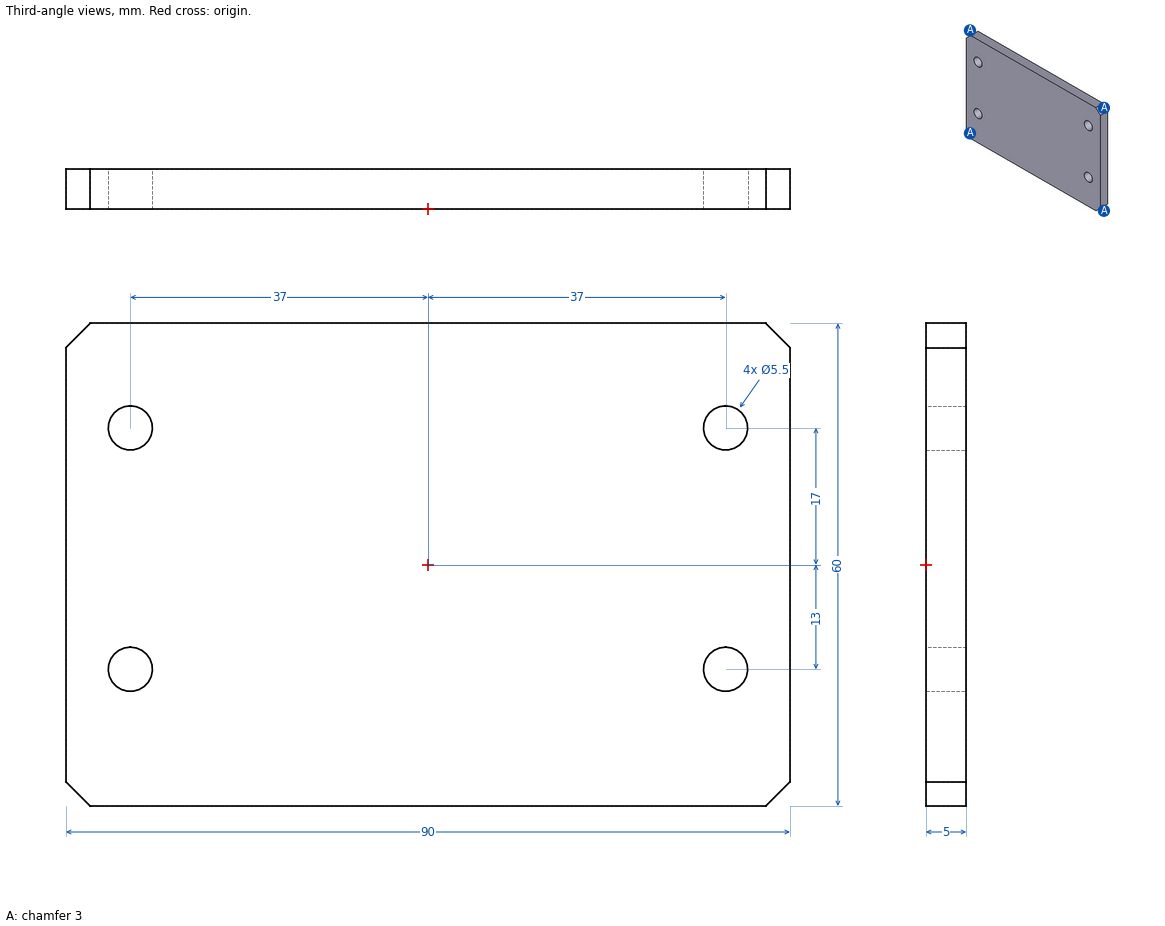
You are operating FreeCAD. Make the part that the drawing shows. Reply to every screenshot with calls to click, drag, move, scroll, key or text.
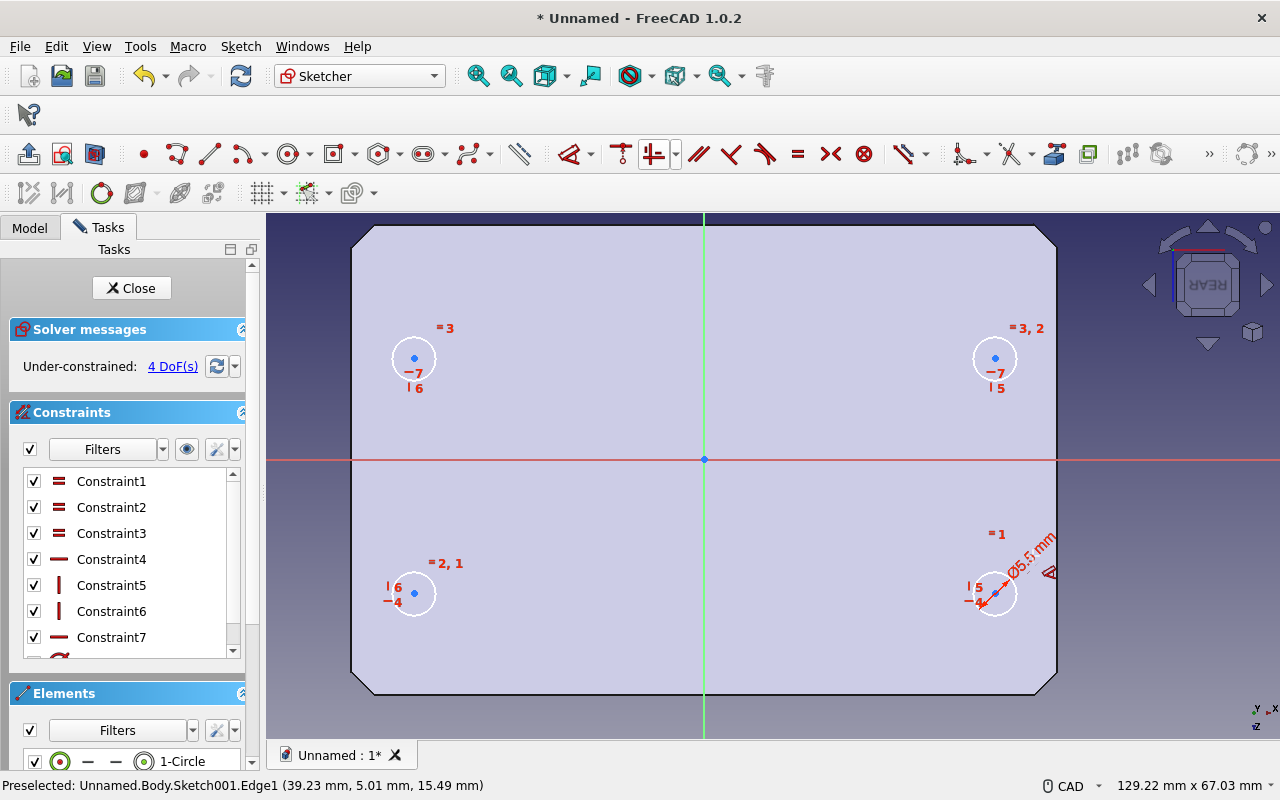
click(995, 594)
click(850, 628)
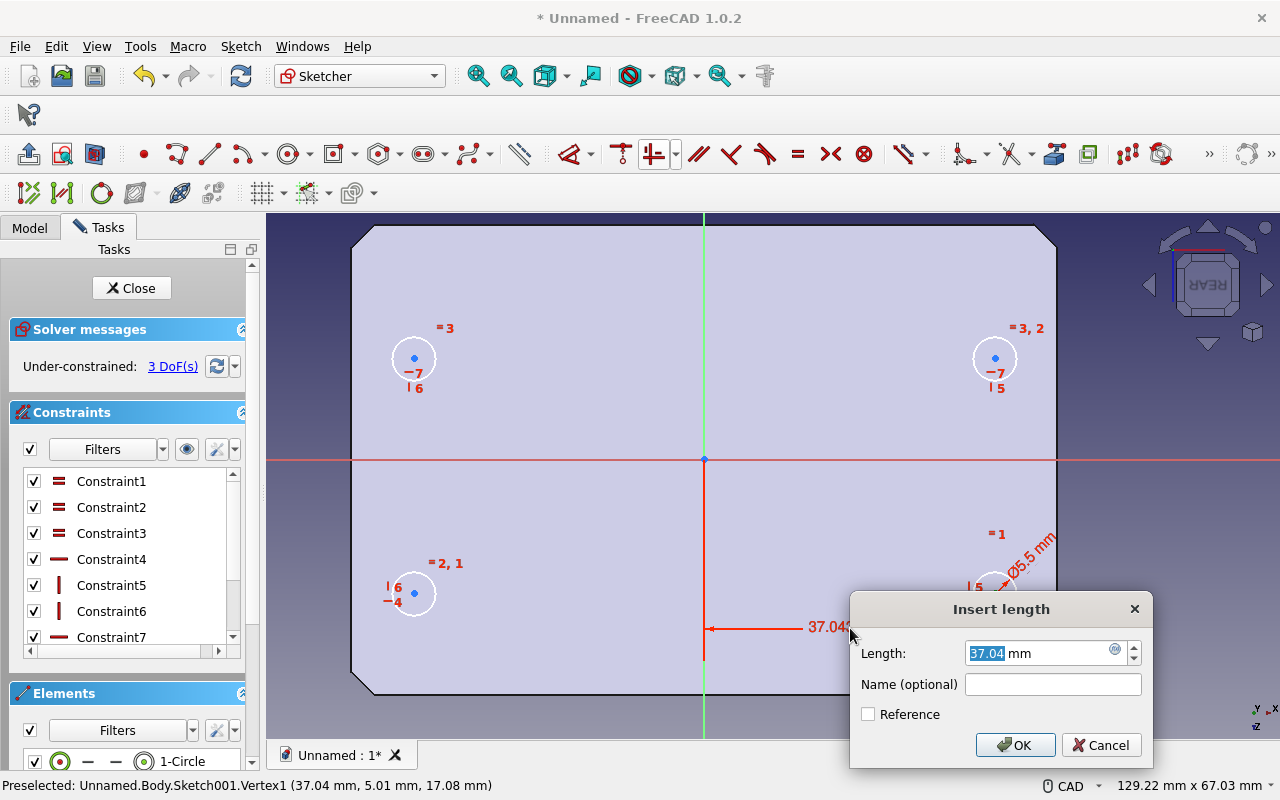
text(37)
key(Return)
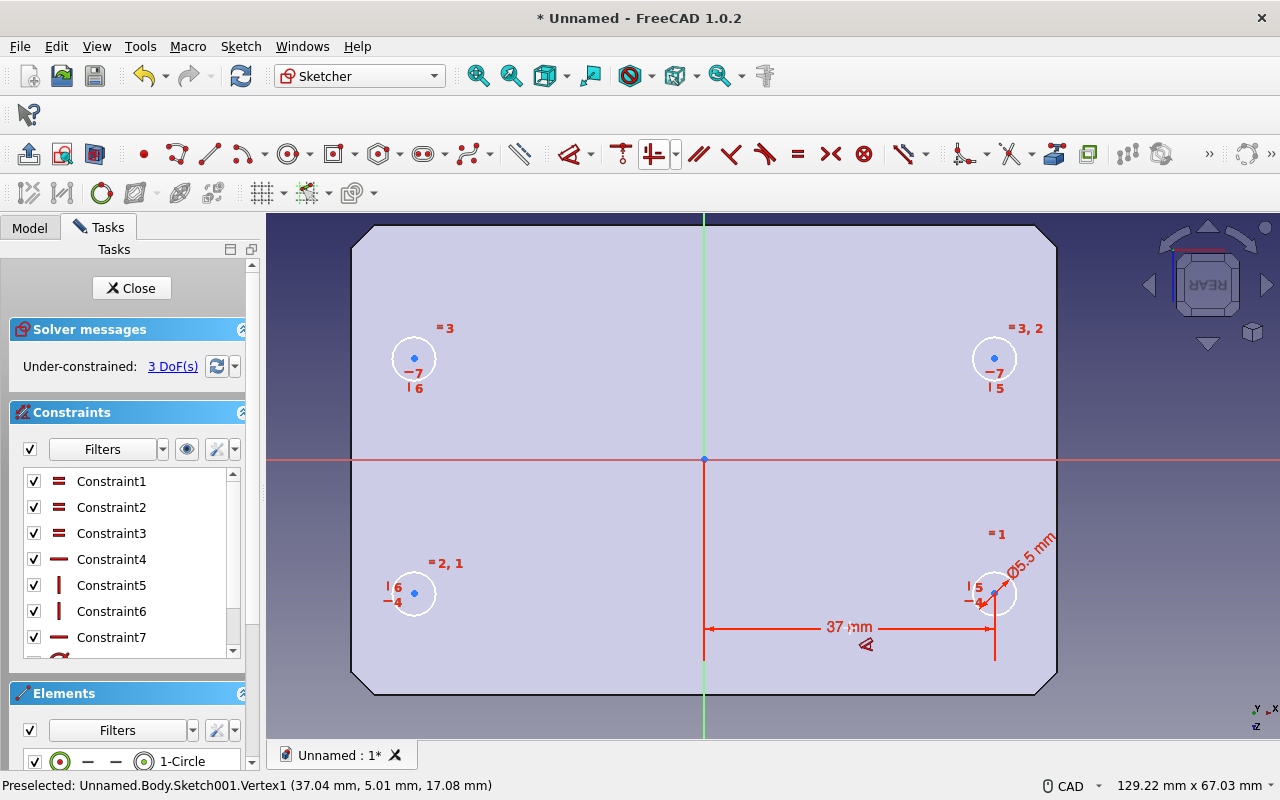
click(995, 594)
click(1029, 527)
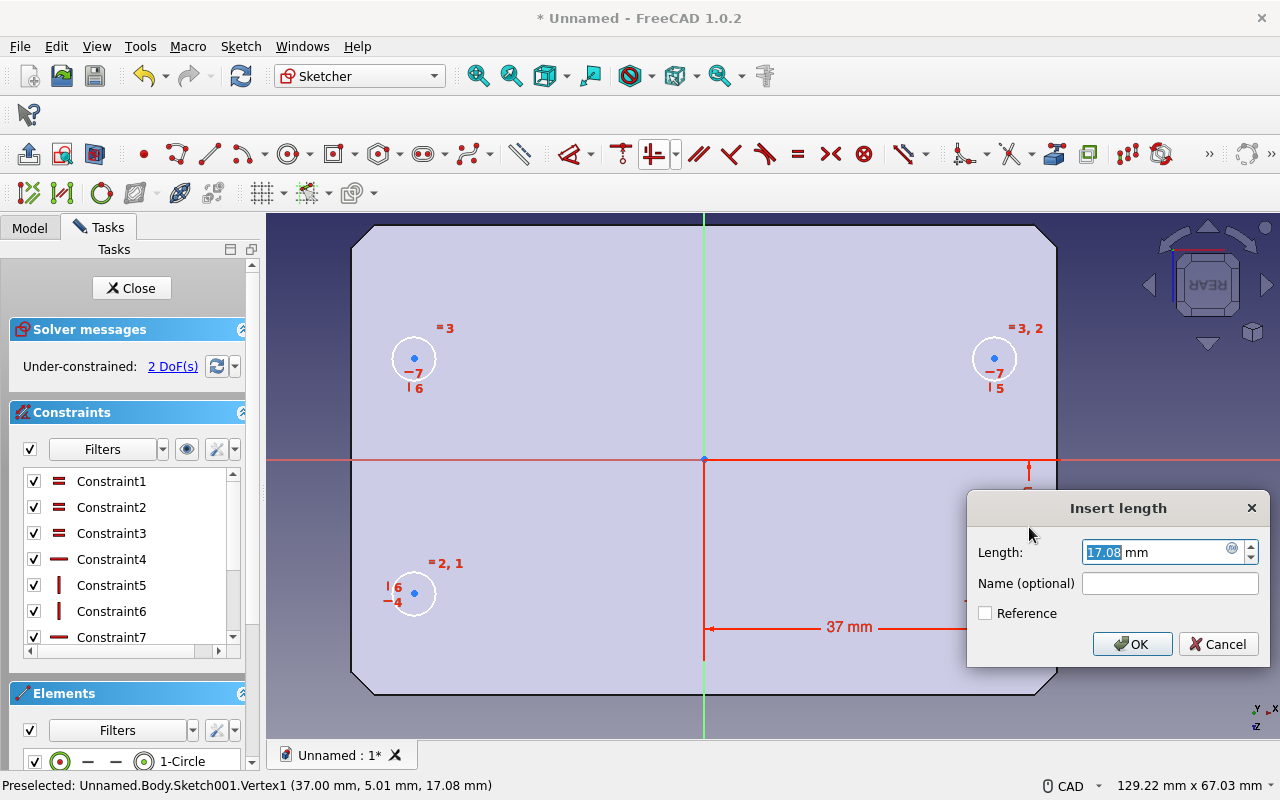
text(17)
key(Return)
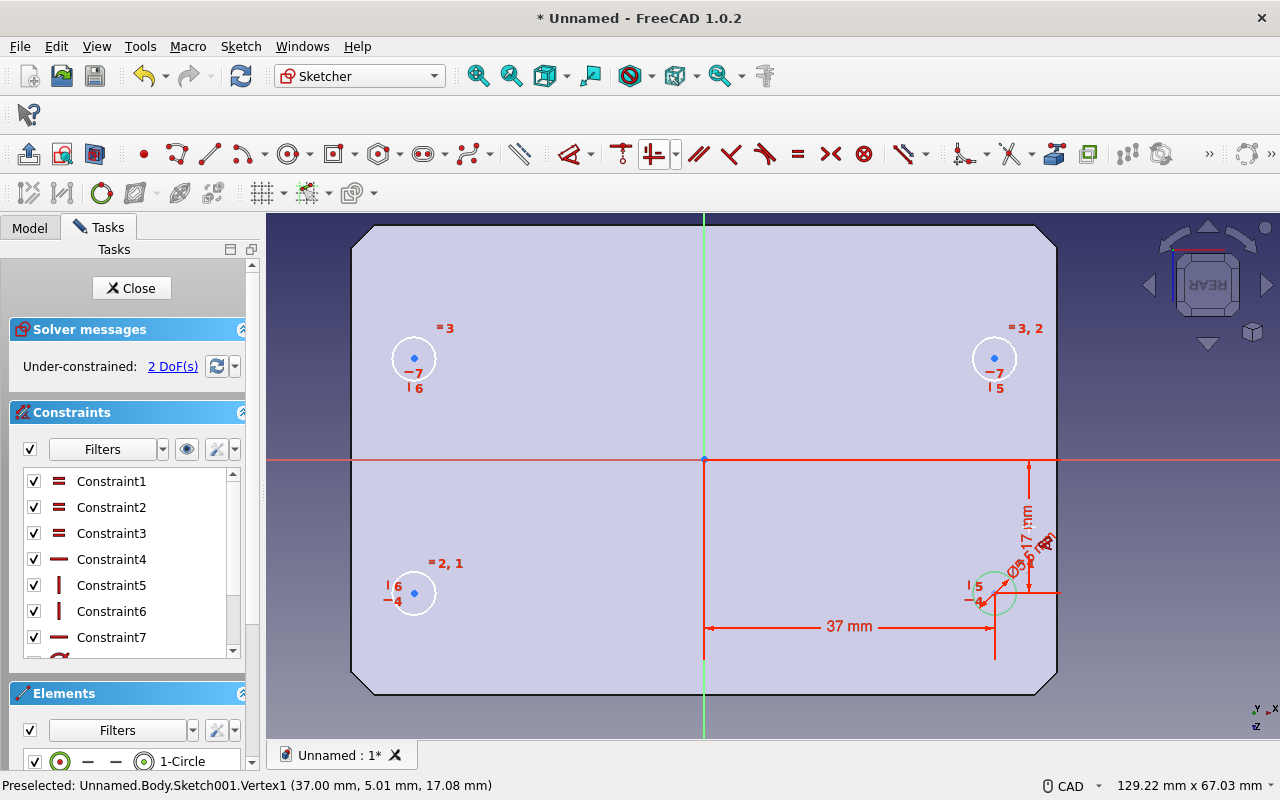
click(414, 593)
click(559, 627)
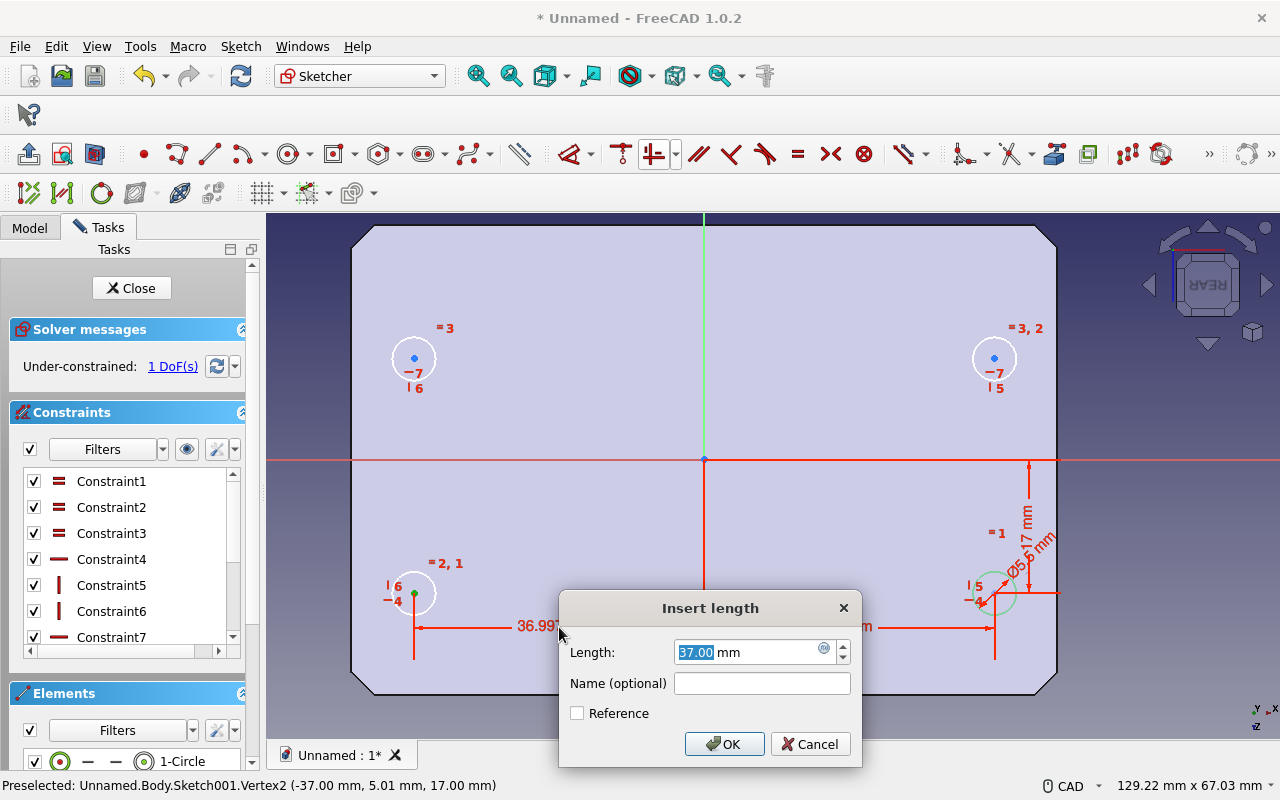
text(37)
key(Return)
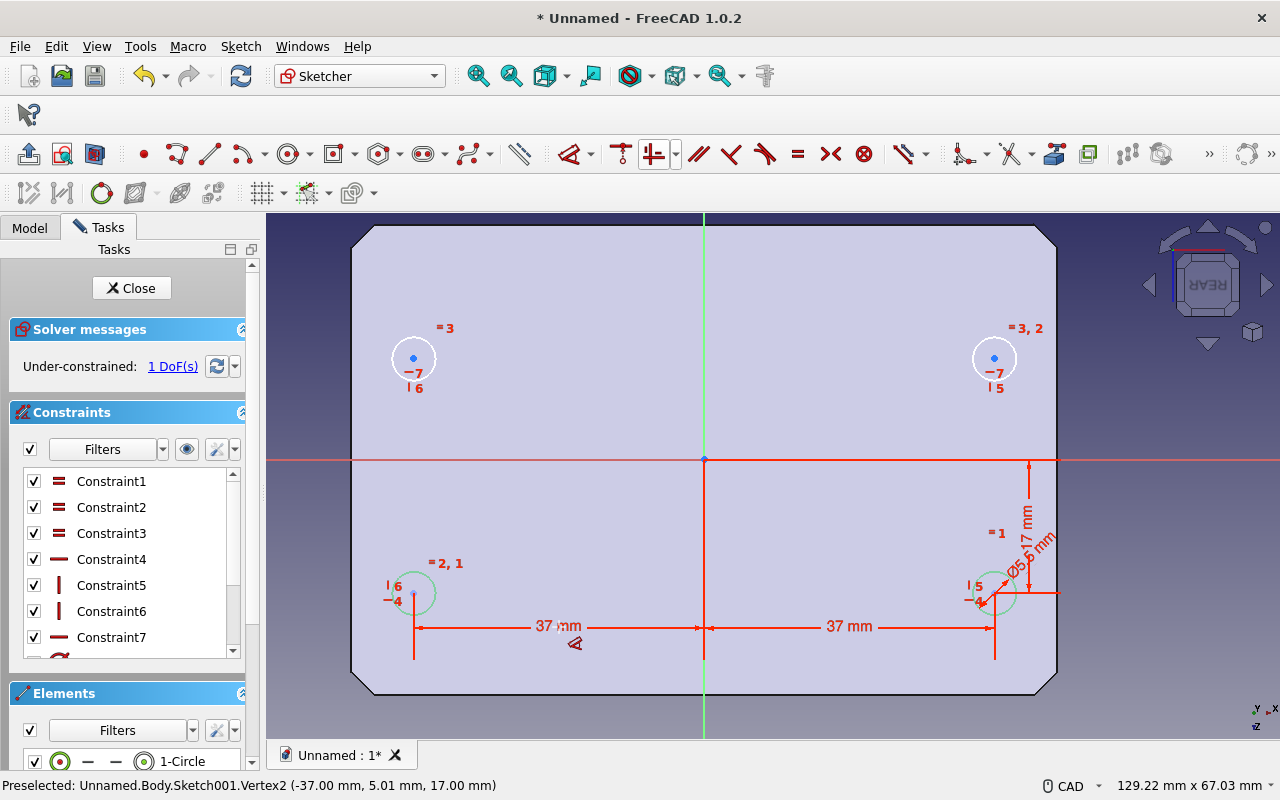
click(995, 359)
click(1029, 409)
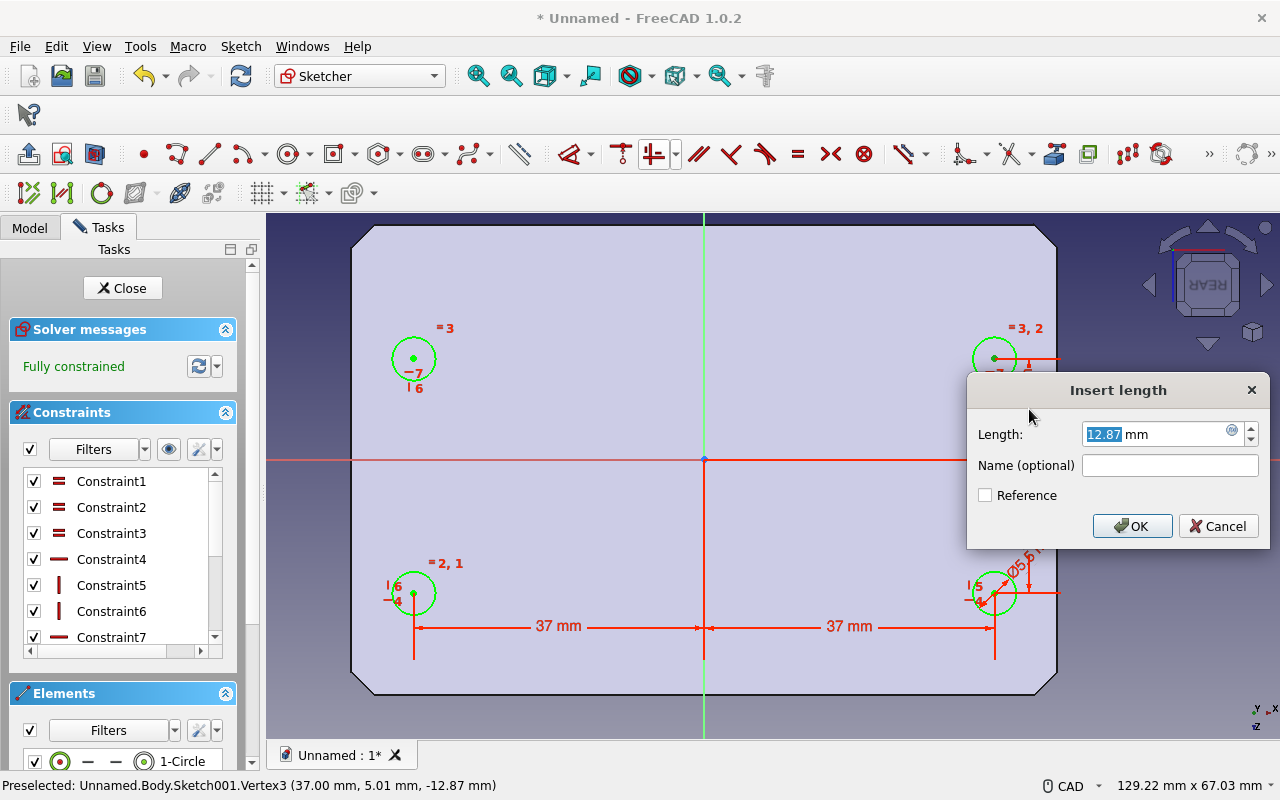
text(13)
key(Return)
key(Escape)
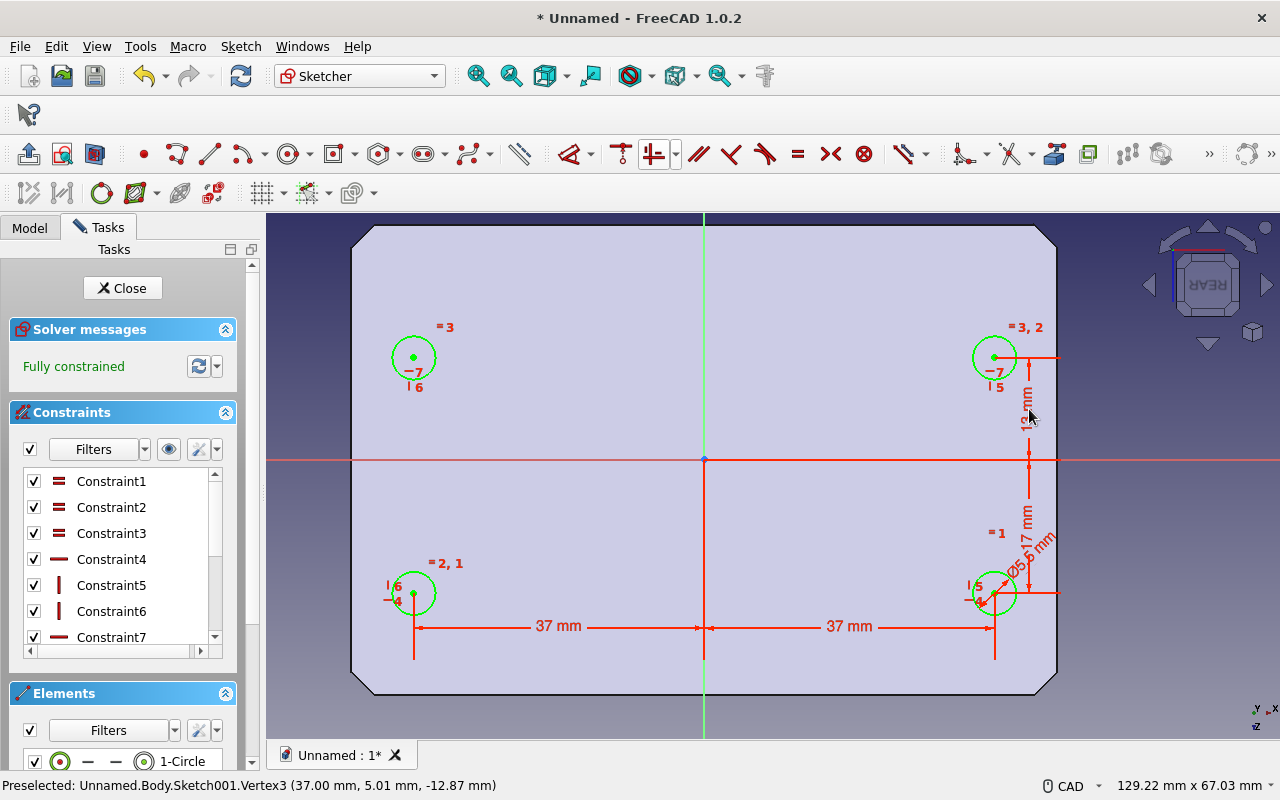
click(123, 288)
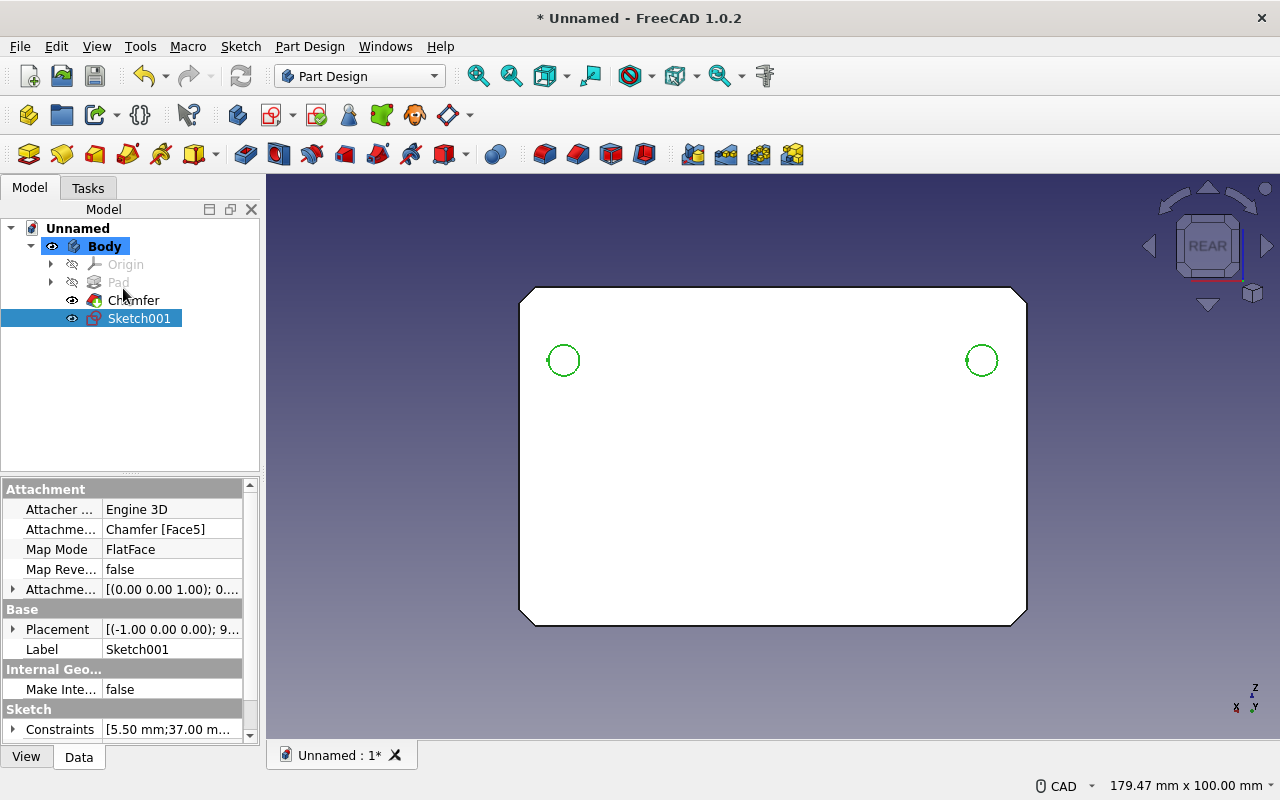
click(246, 154)